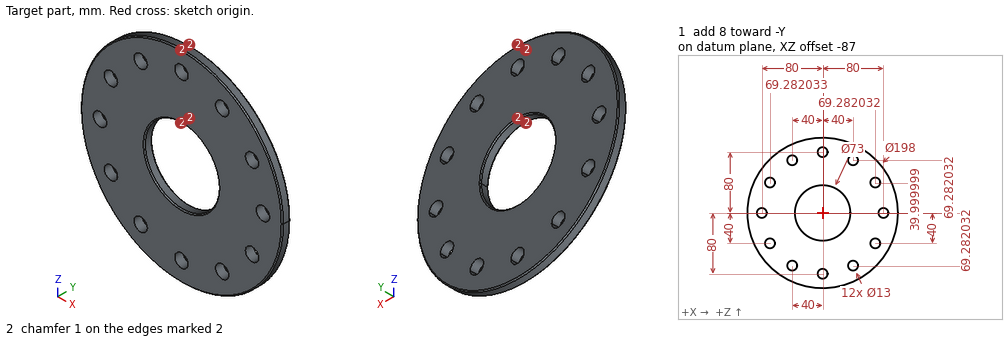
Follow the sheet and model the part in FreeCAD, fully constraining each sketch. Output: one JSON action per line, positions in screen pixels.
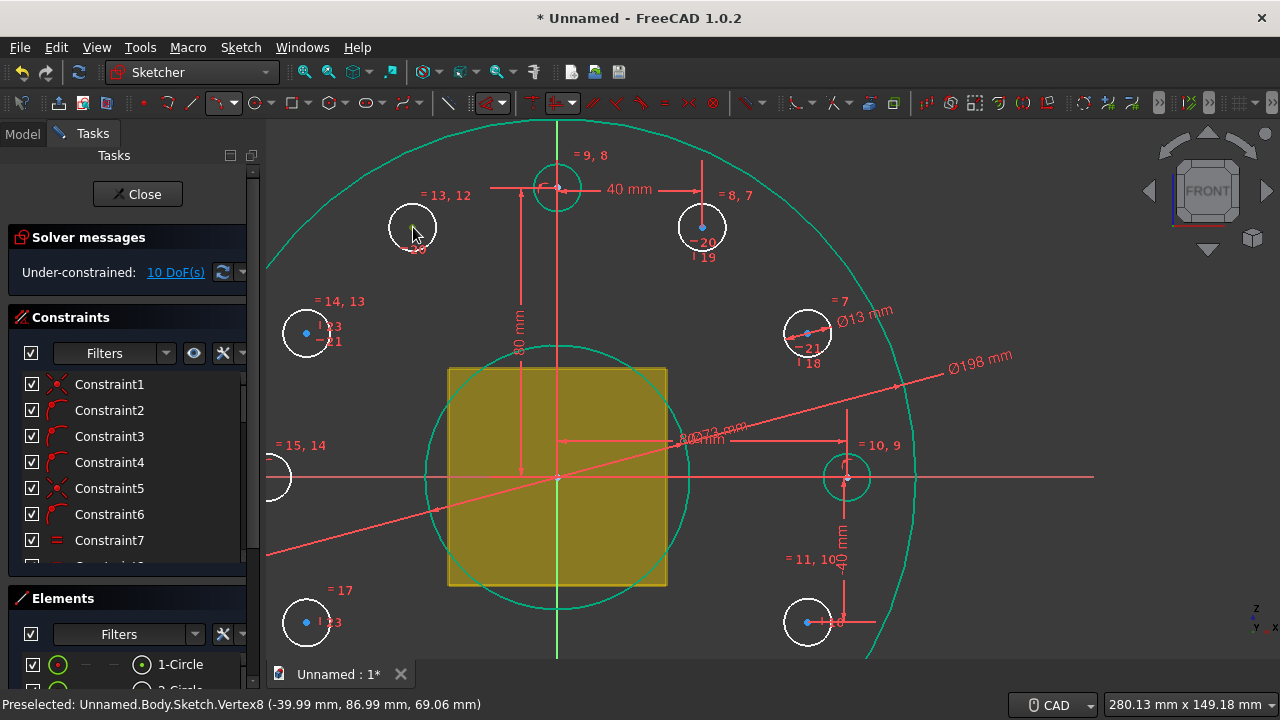
{"action": "key", "text": "l"}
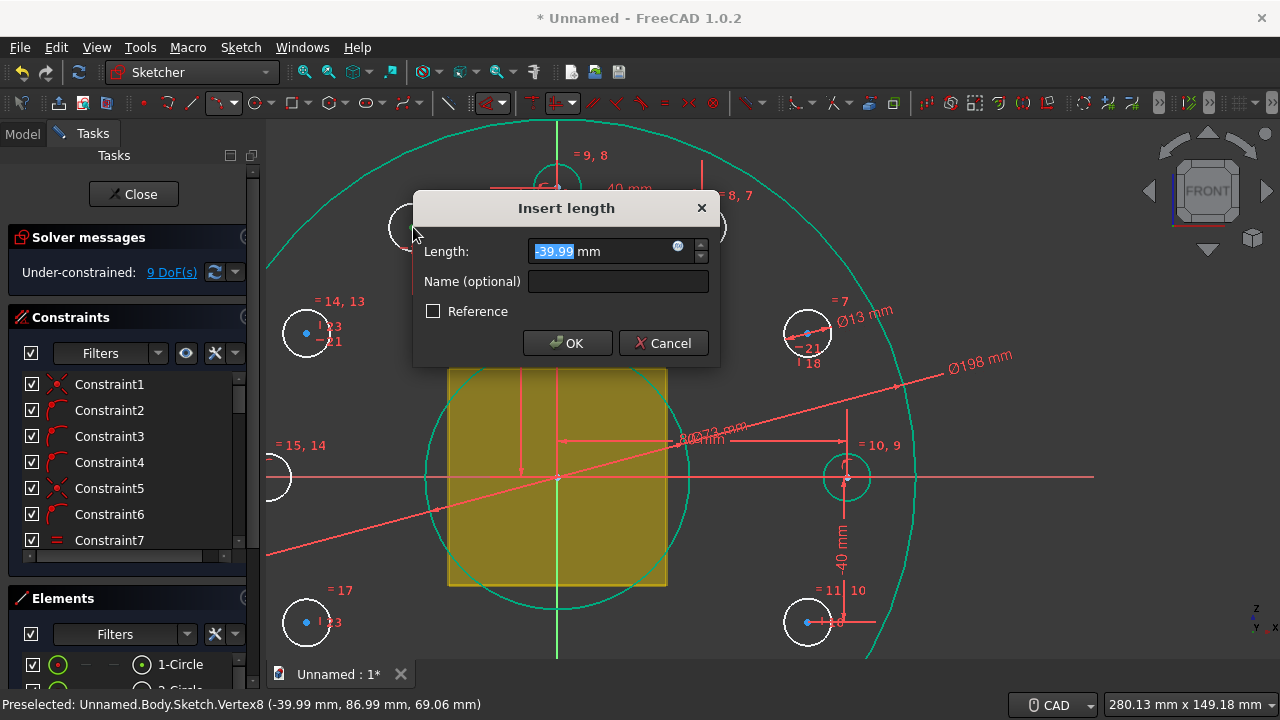
{"action": "type", "text": "-40"}
{"action": "key", "text": "Return"}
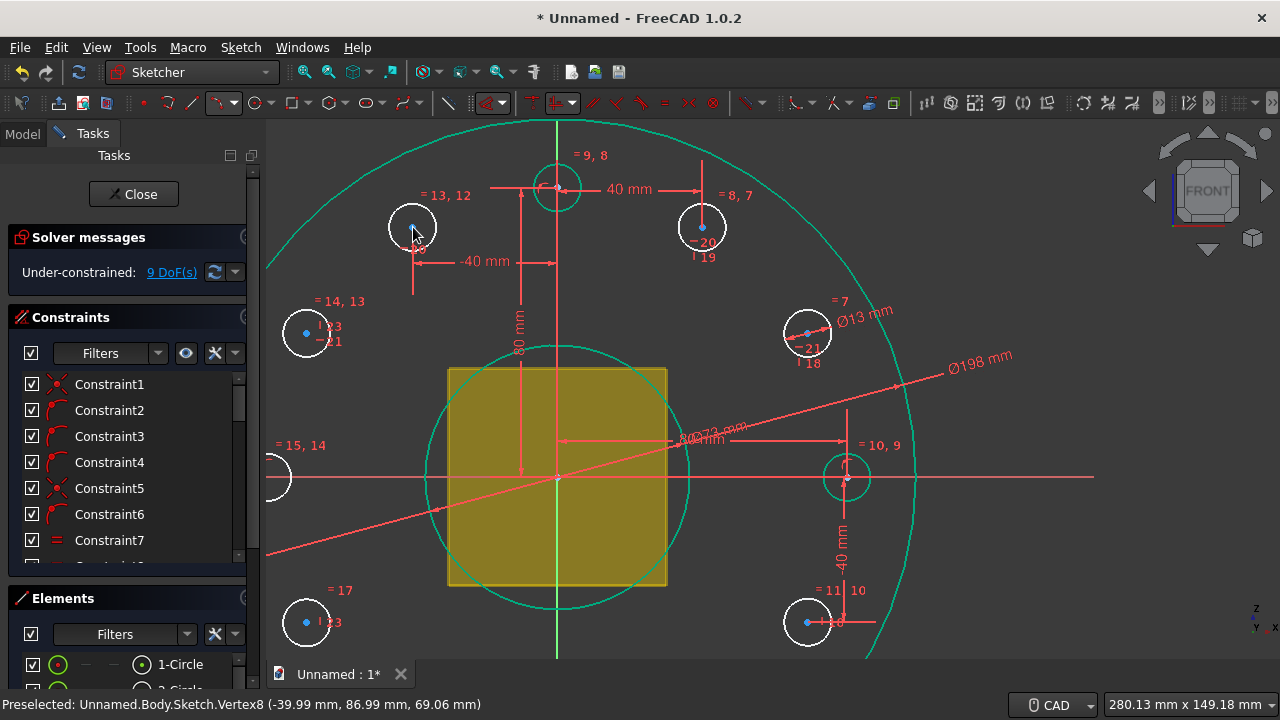
{"action": "scroll", "coordinate": [825, 317], "scroll_direction": "down", "scroll_amount": 4}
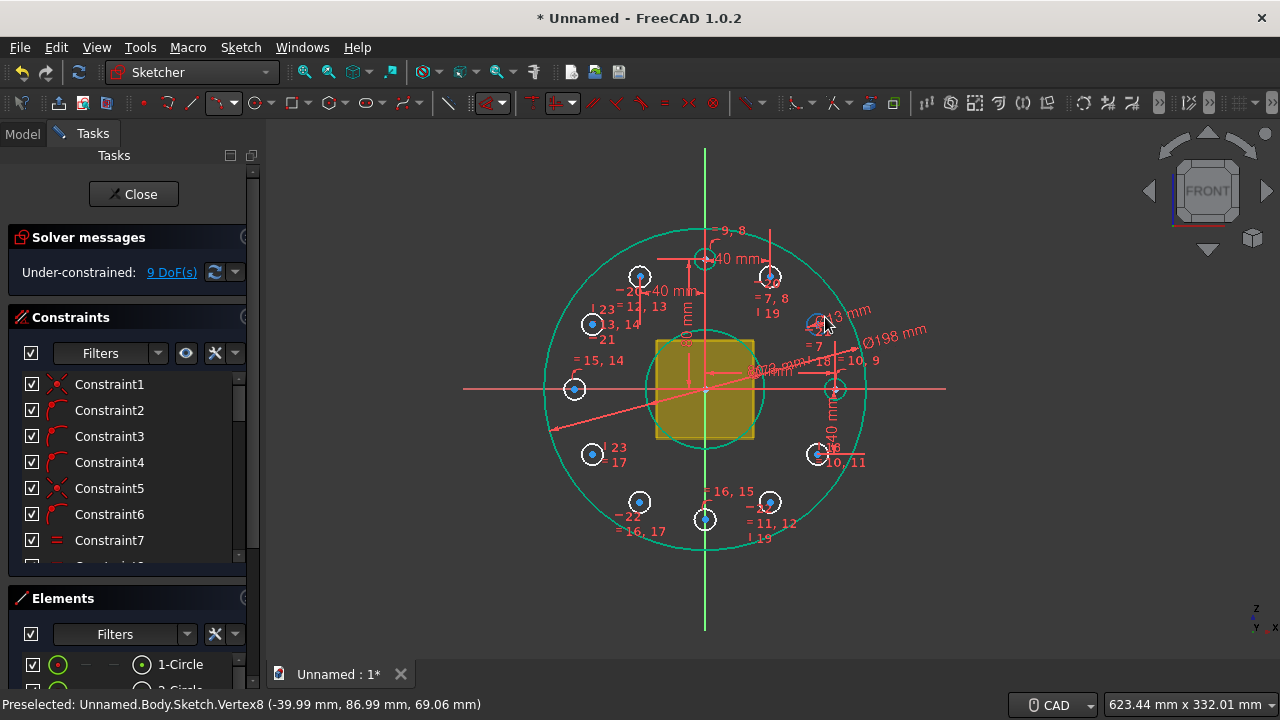
{"action": "left_click", "coordinate": [575, 389]}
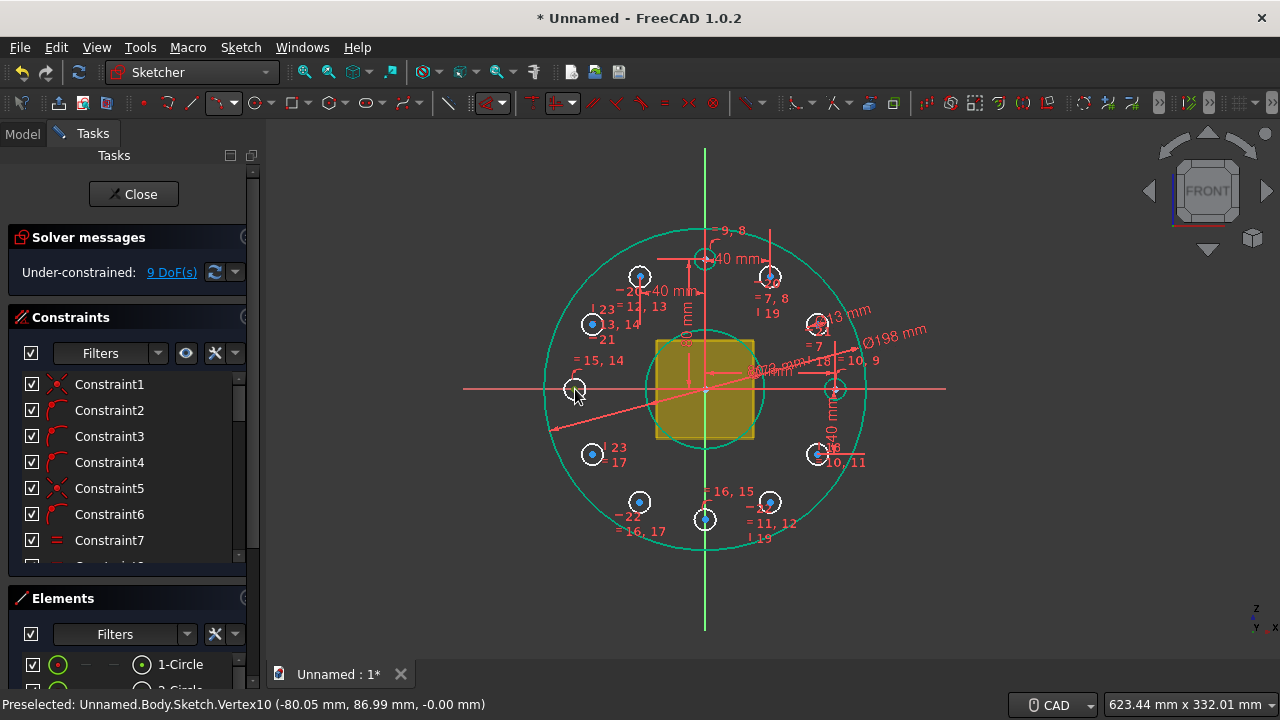
{"action": "key", "text": "l"}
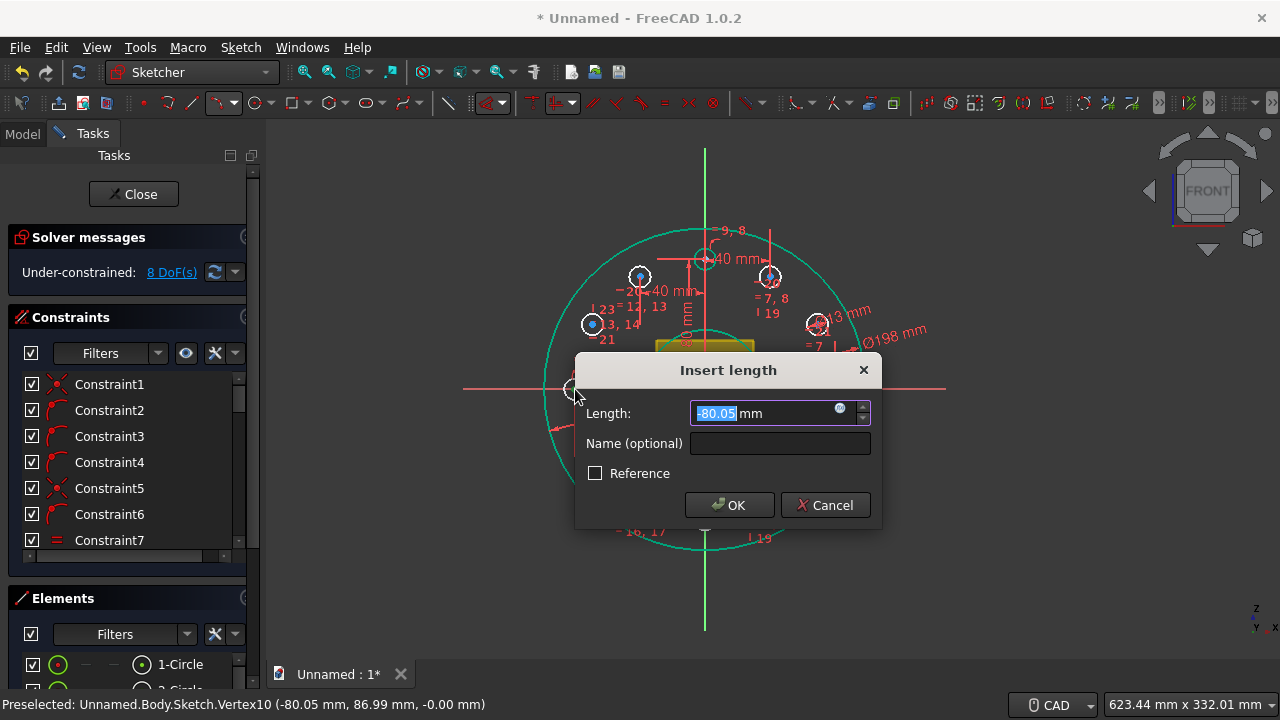
{"action": "type", "text": "-80"}
{"action": "key", "text": "Return"}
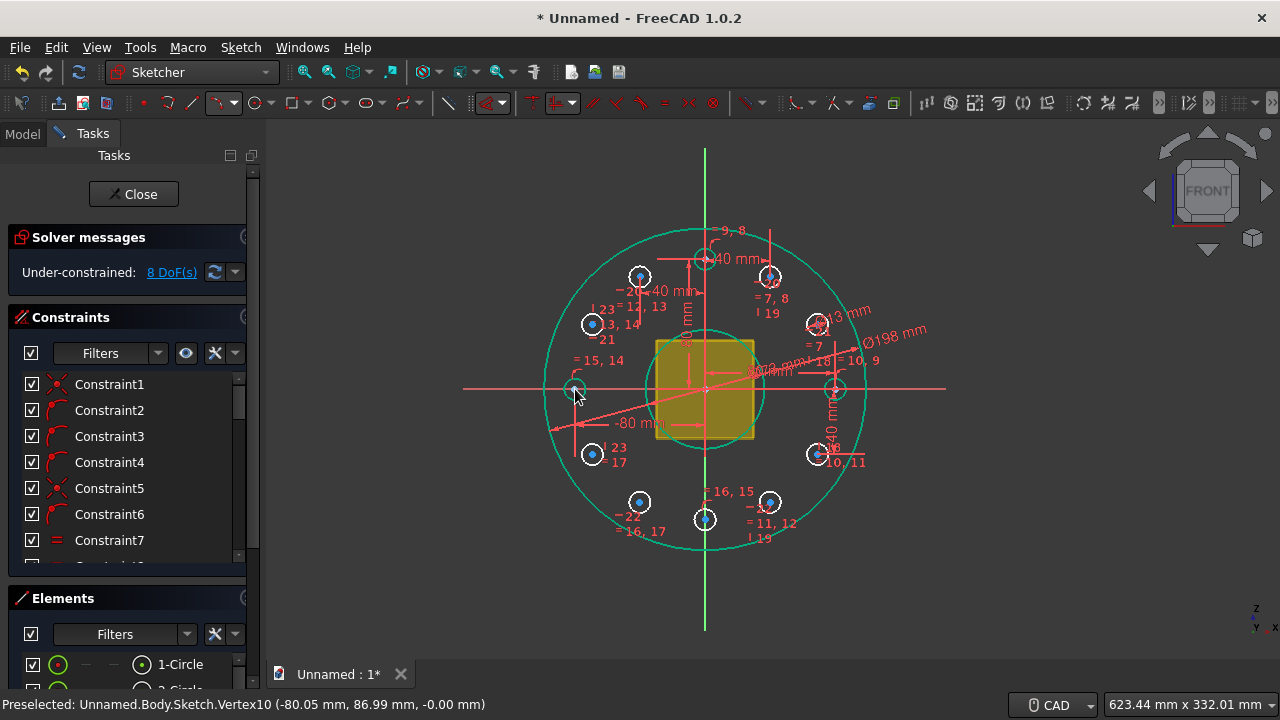
{"action": "left_click", "coordinate": [705, 520]}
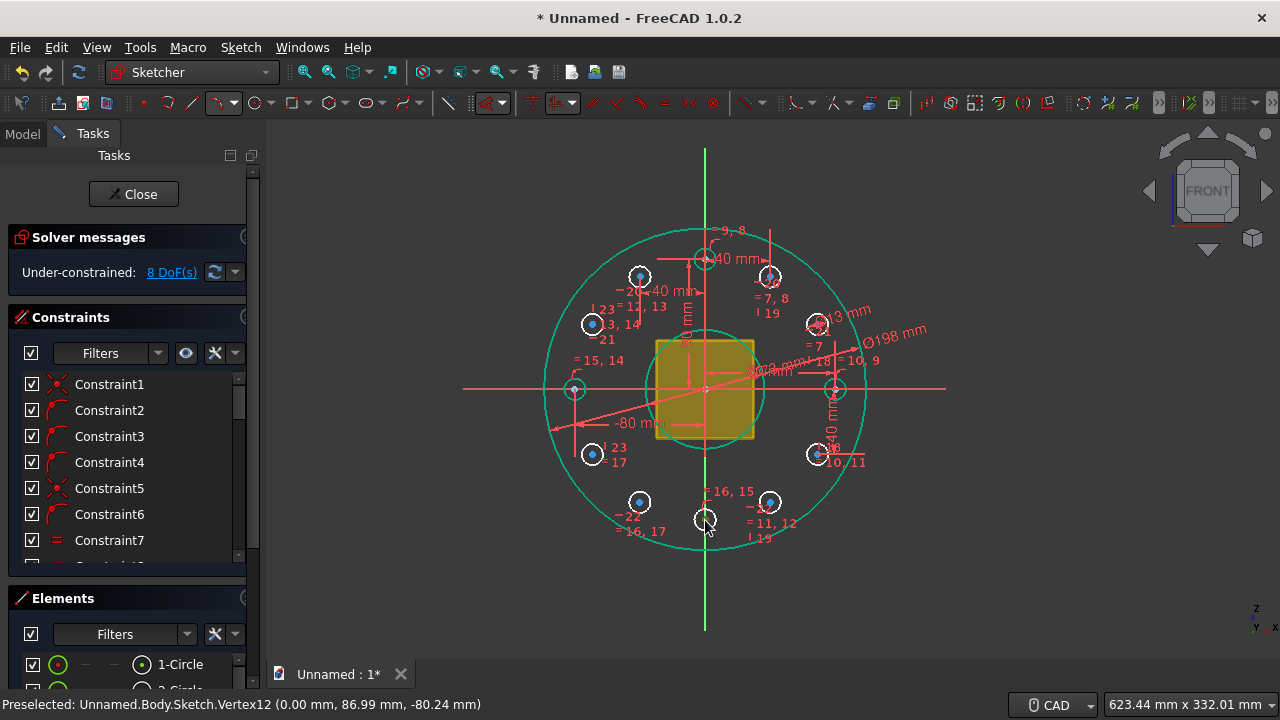
{"action": "left_click", "coordinate": [504, 104]}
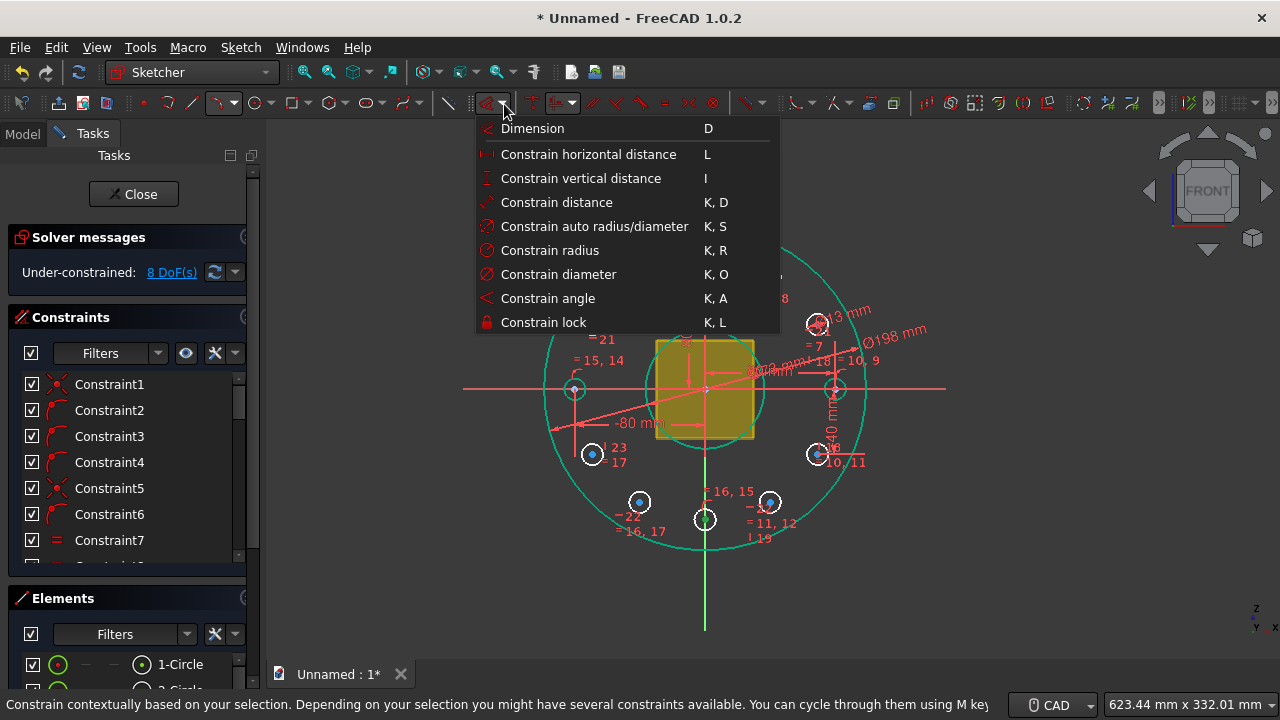
{"action": "left_click", "coordinate": [628, 178]}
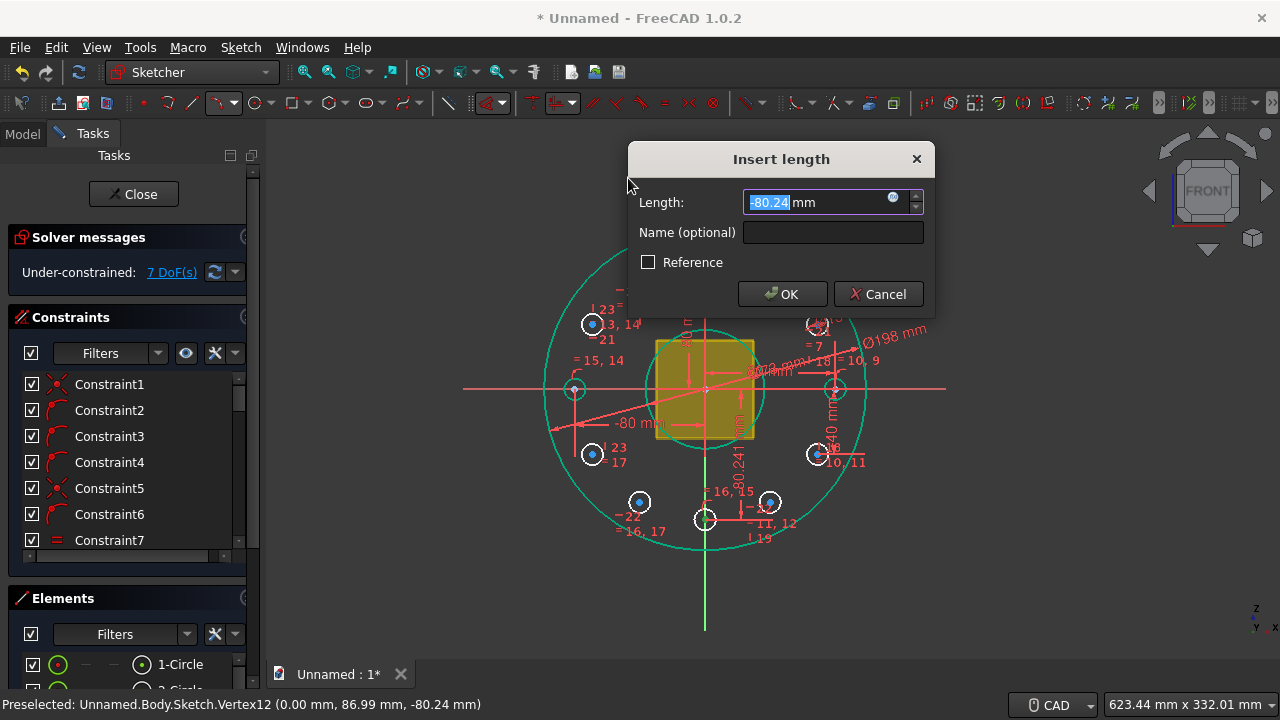
{"action": "type", "text": "-80"}
{"action": "key", "text": "Return"}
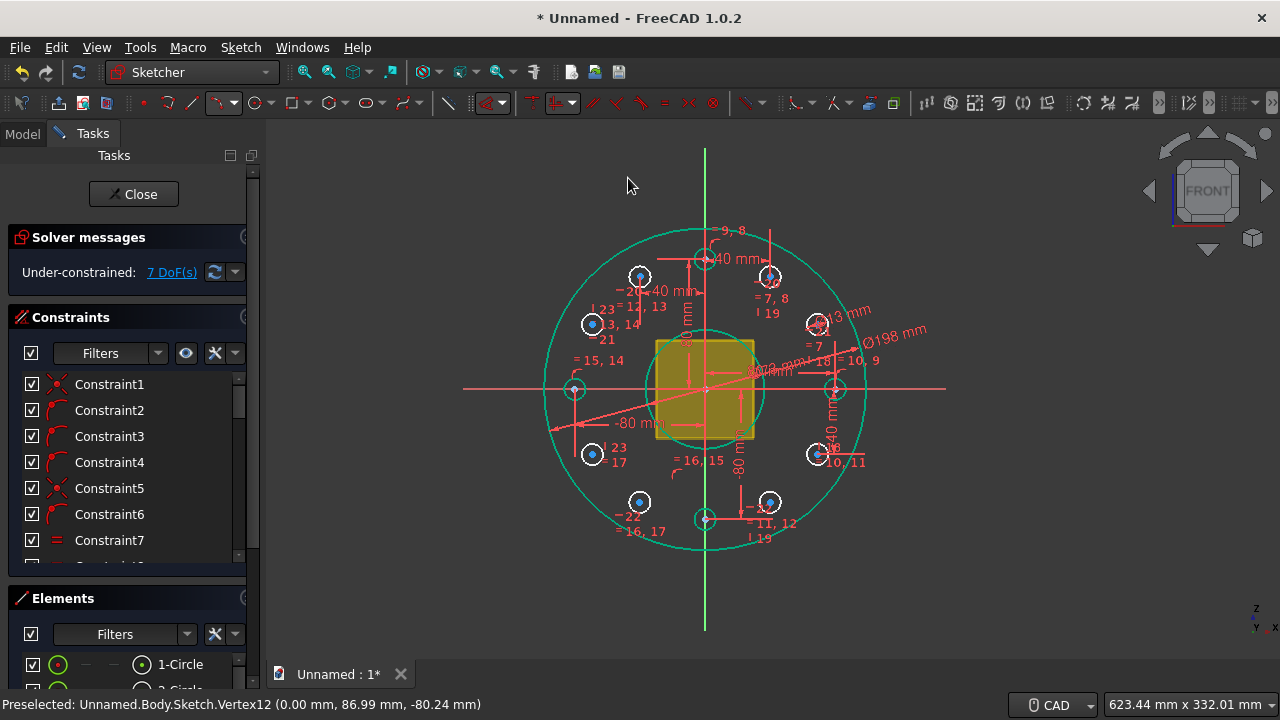
{"action": "left_click", "coordinate": [640, 502]}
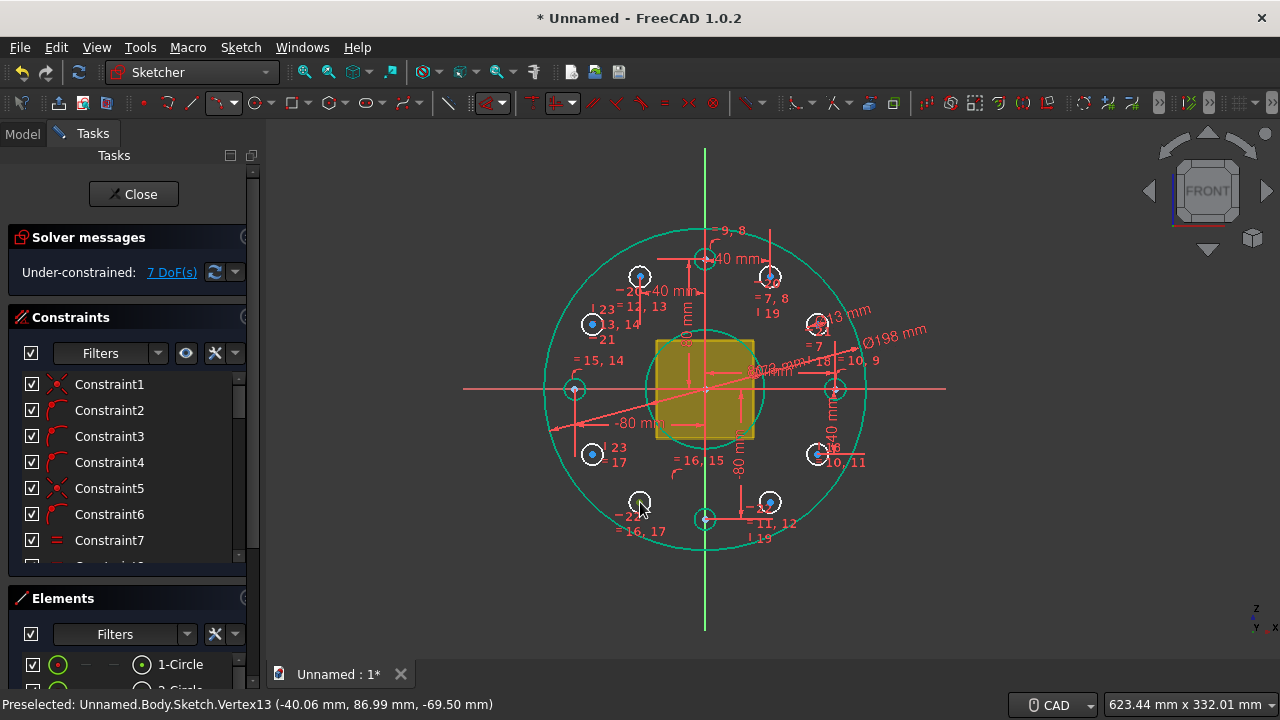
{"action": "key", "text": "l"}